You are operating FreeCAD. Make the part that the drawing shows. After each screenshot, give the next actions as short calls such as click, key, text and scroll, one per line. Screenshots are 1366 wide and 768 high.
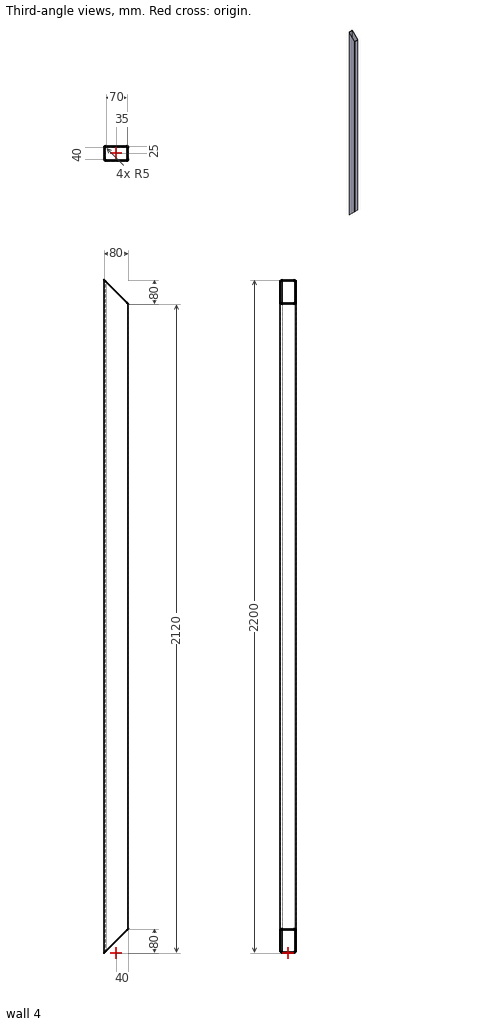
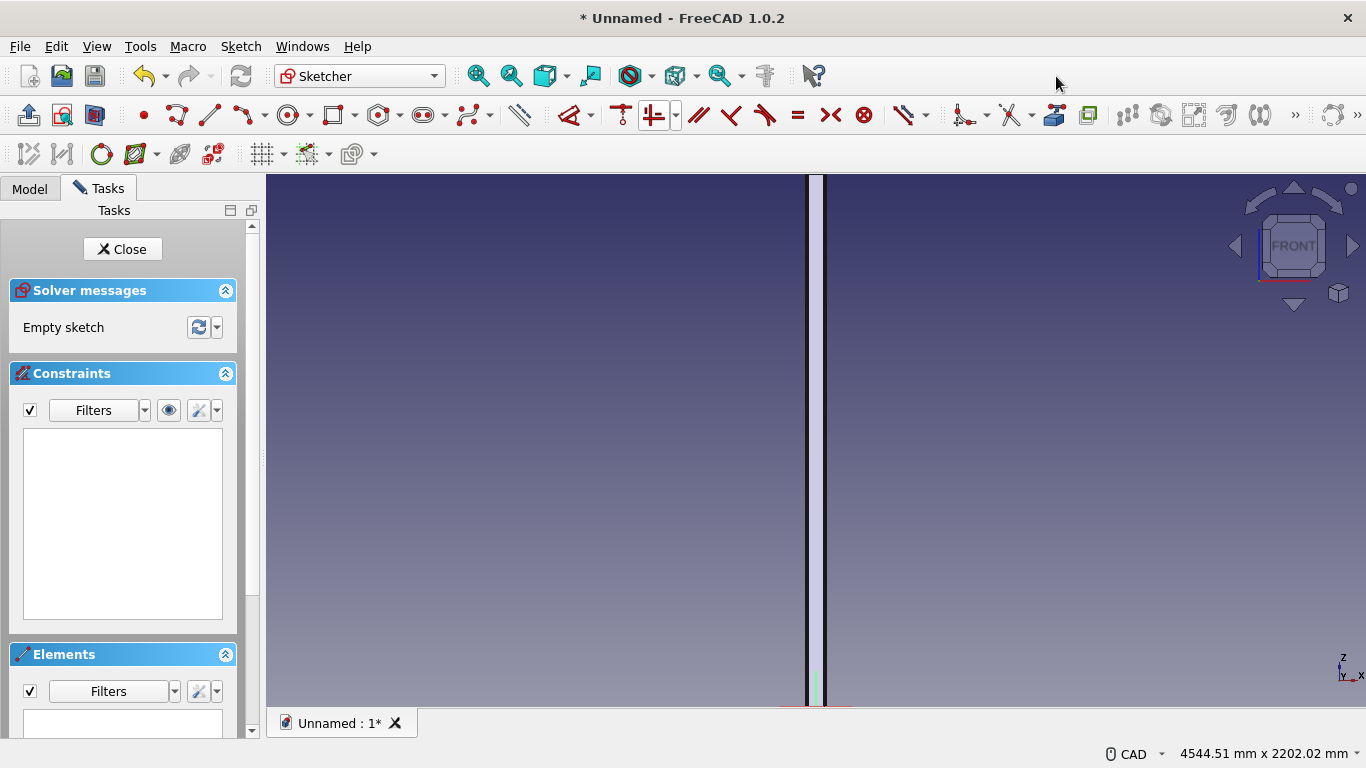
scroll(608, 441, down, 2)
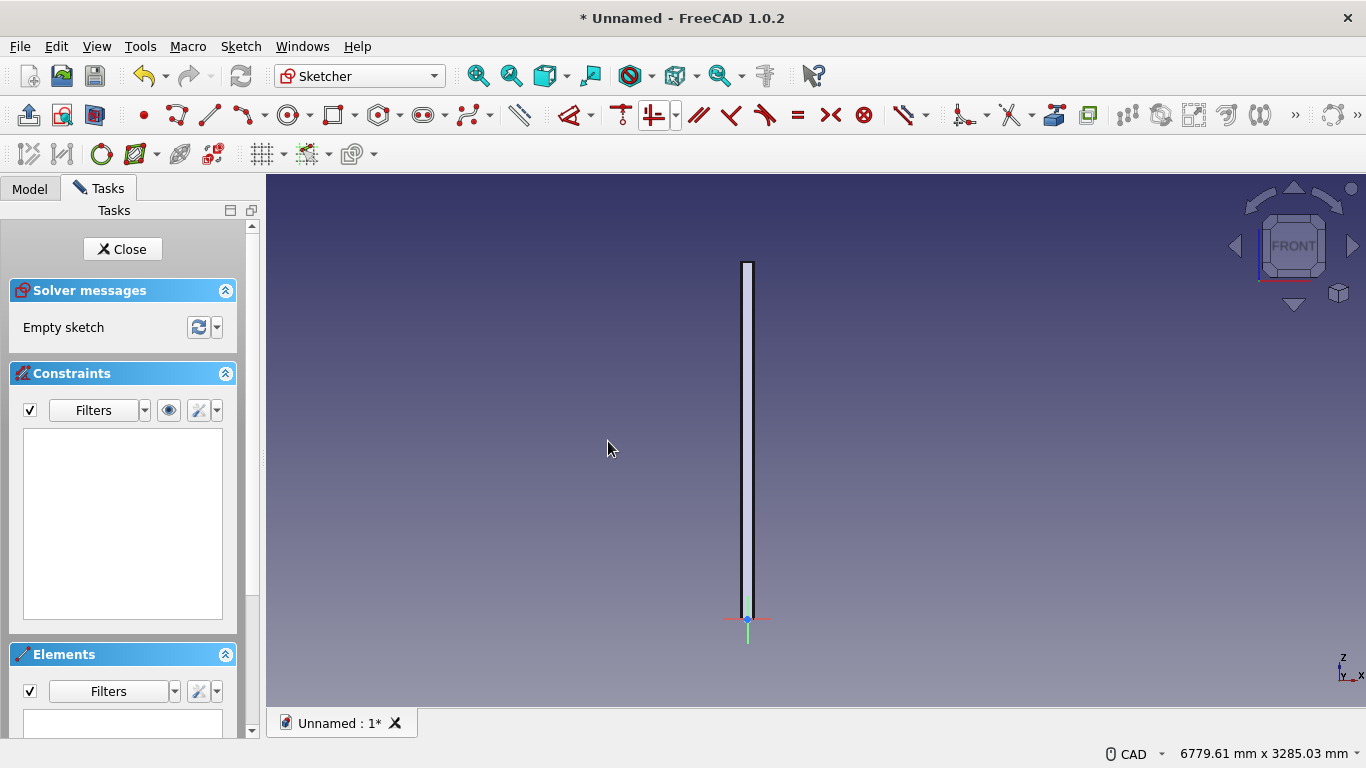
click(177, 116)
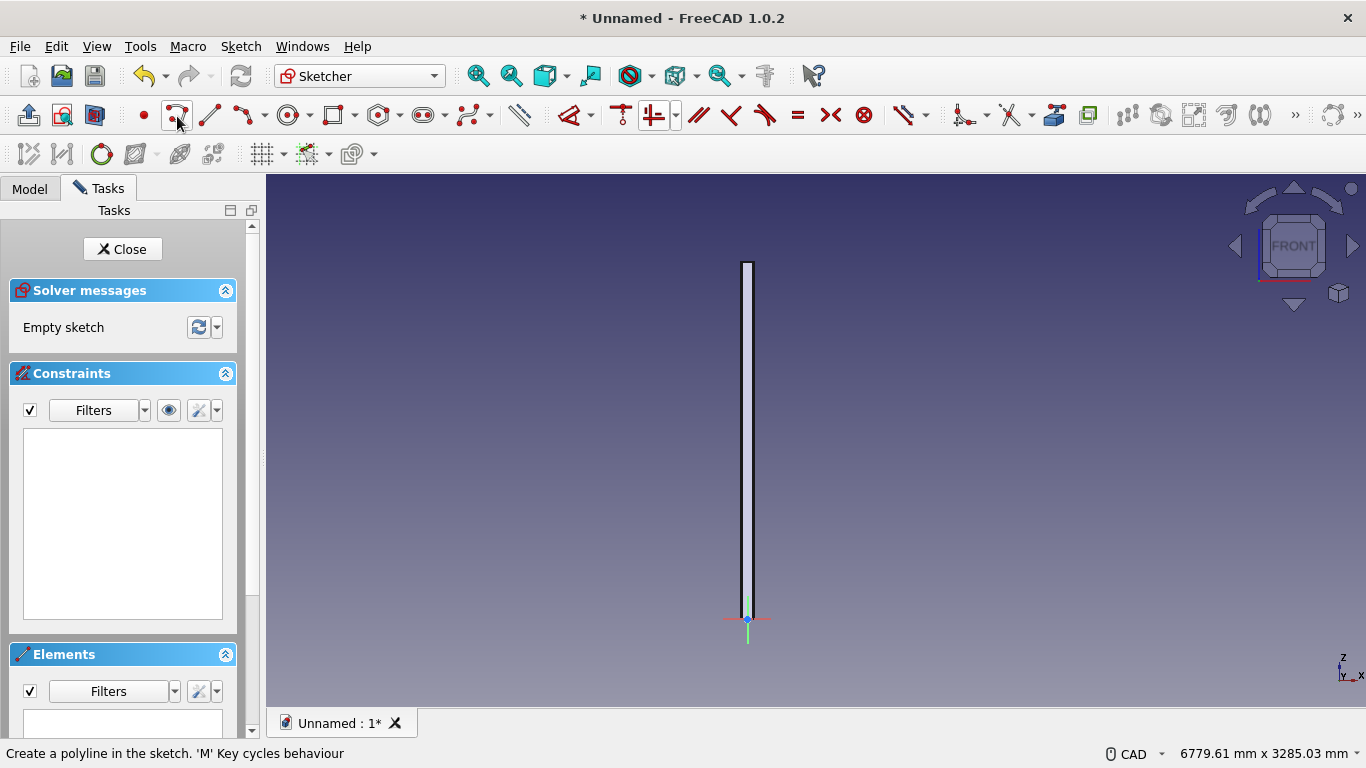
scroll(754, 275, up, 5)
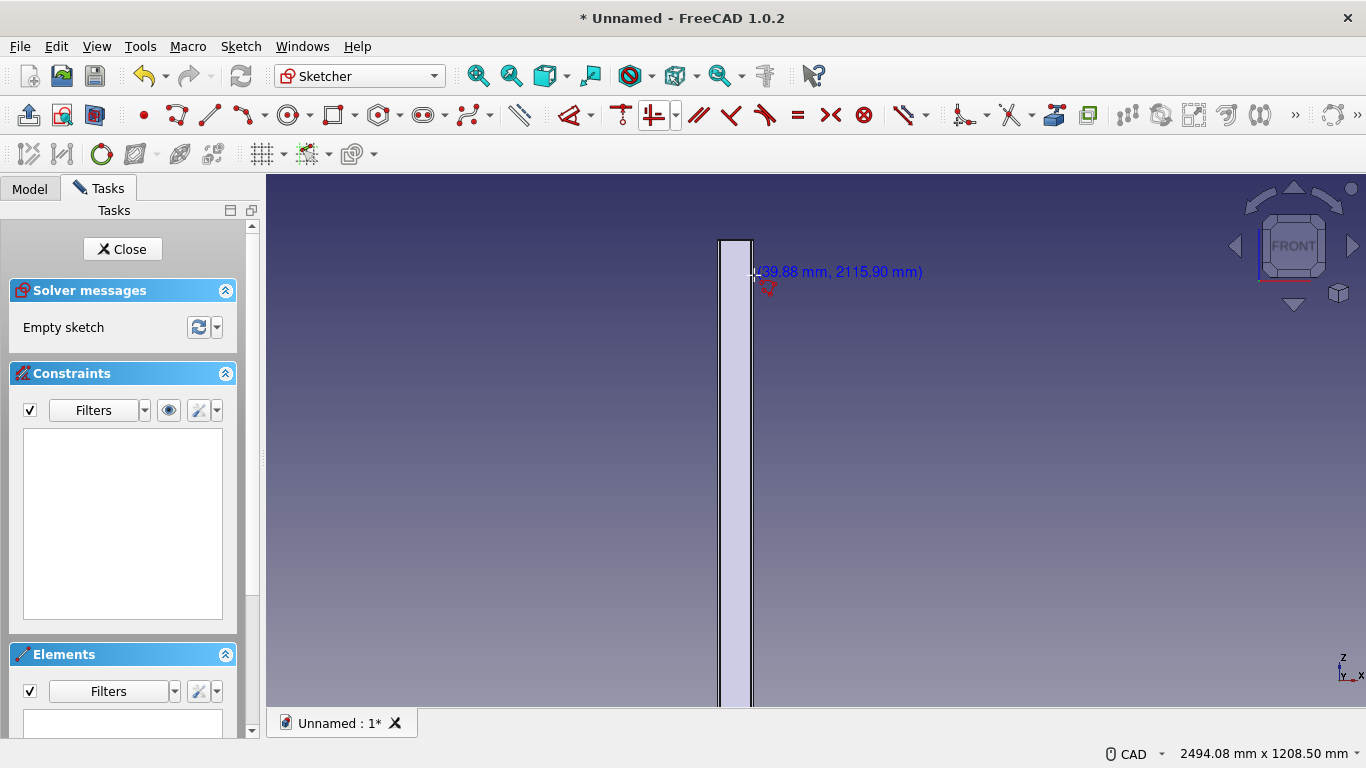
click(753, 276)
click(753, 240)
click(718, 240)
click(753, 277)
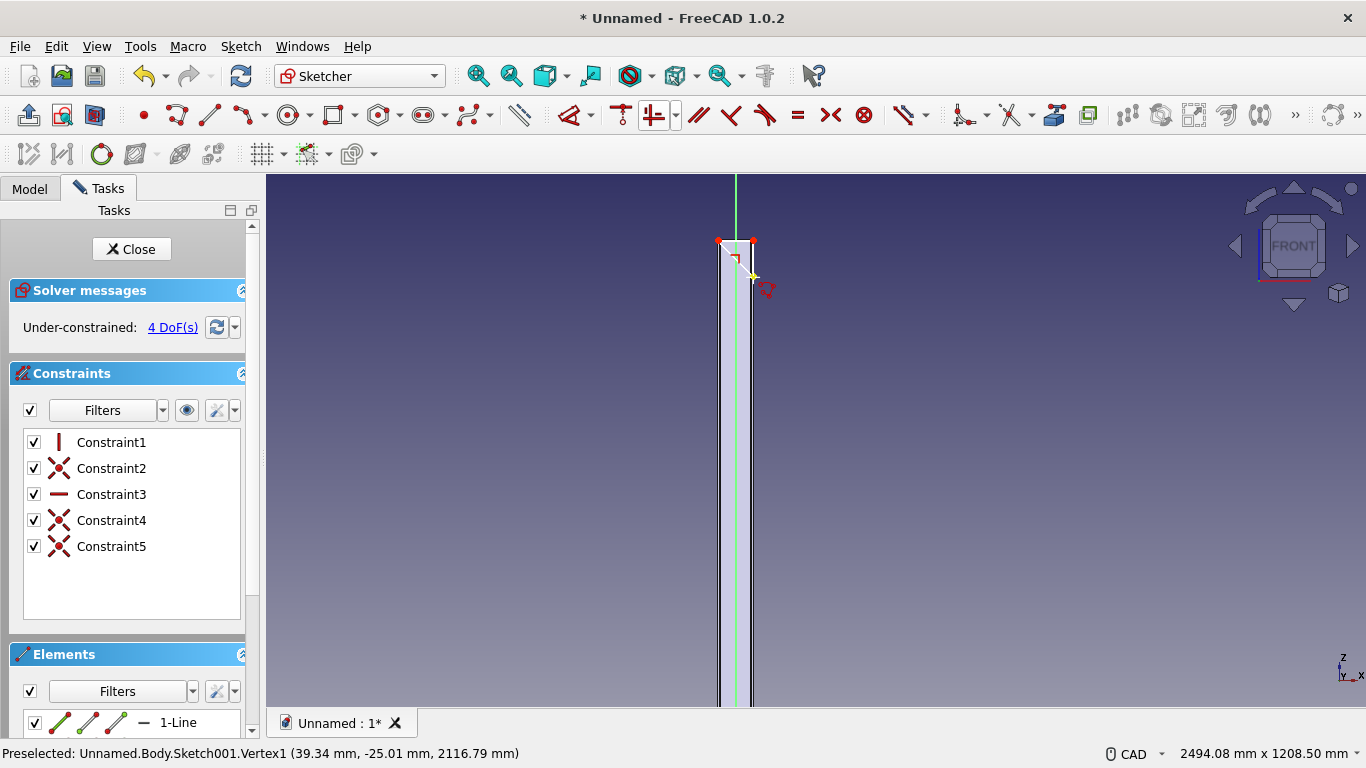
scroll(754, 275, down, 5)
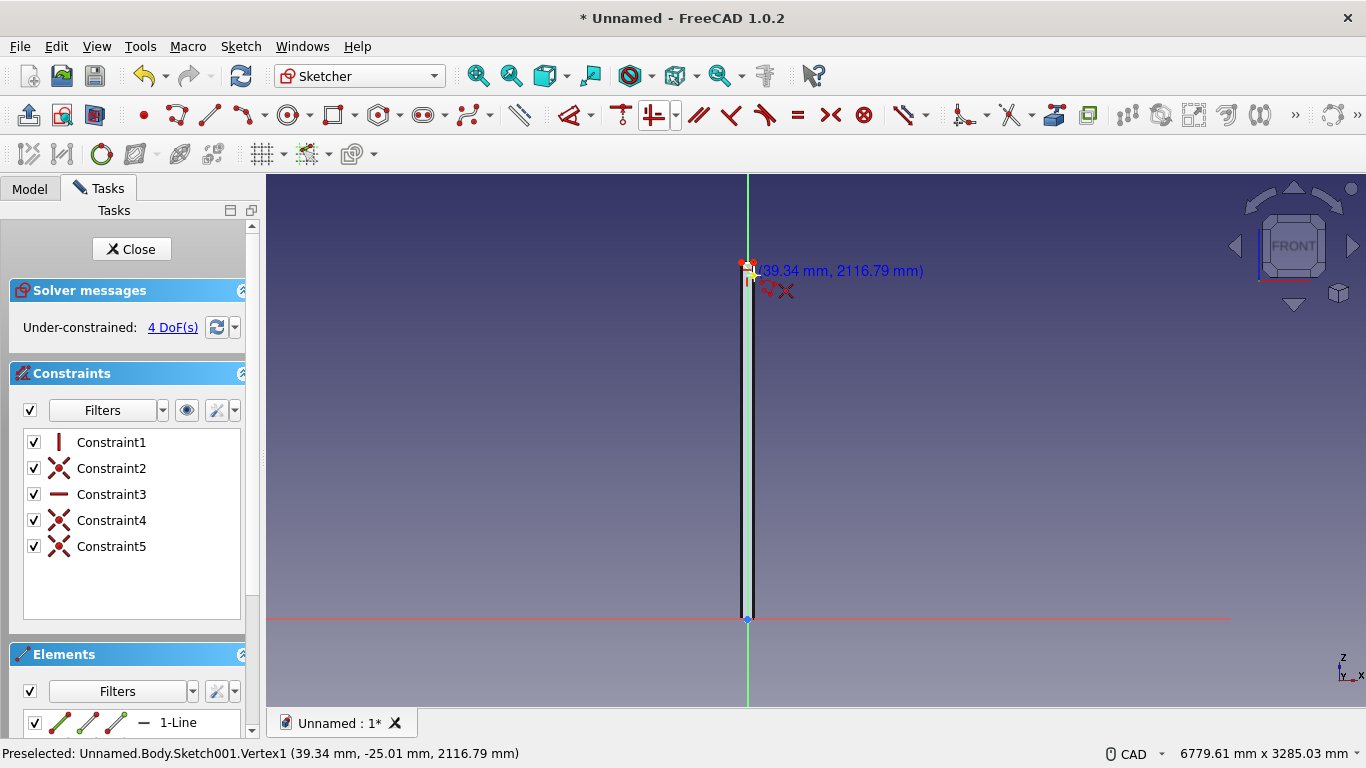
scroll(754, 619, up, 5)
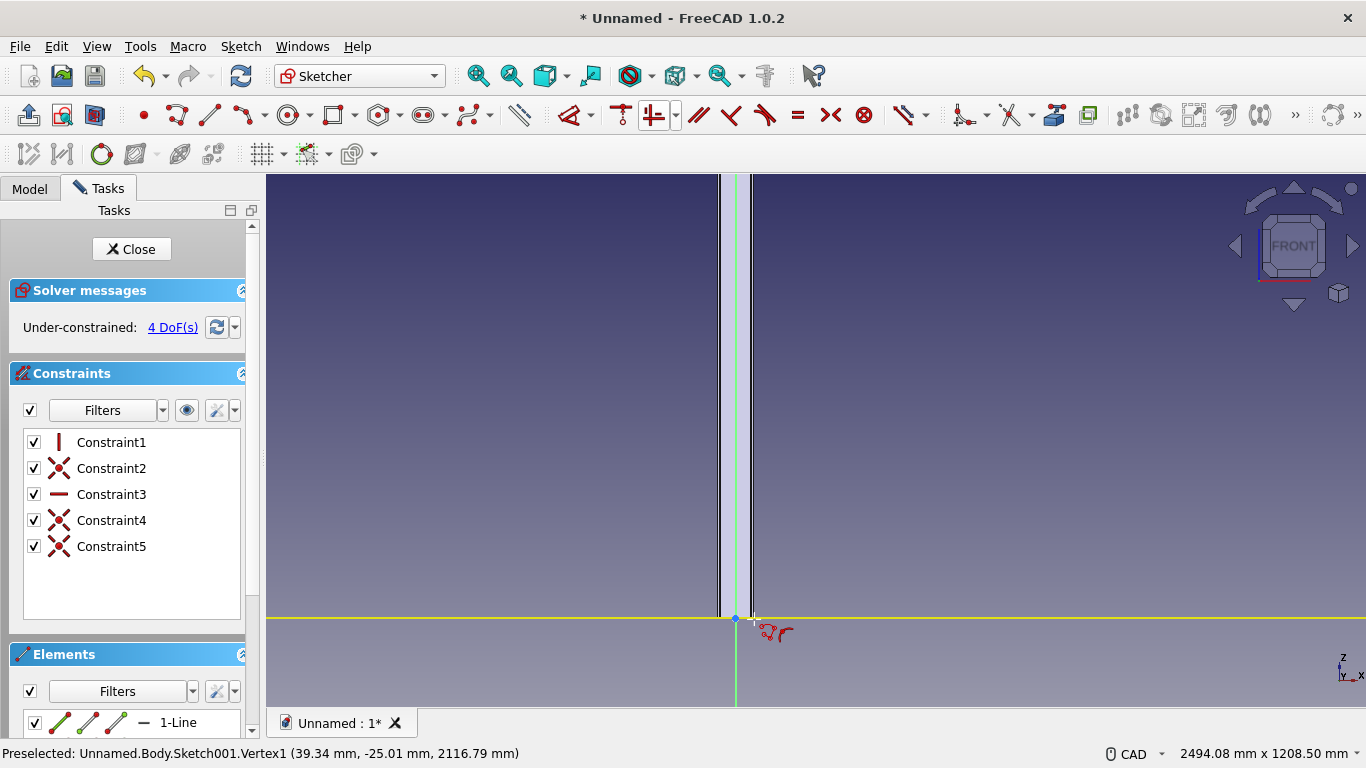
click(753, 618)
click(753, 583)
click(718, 609)
click(753, 618)
key(Escape)
key(Escape)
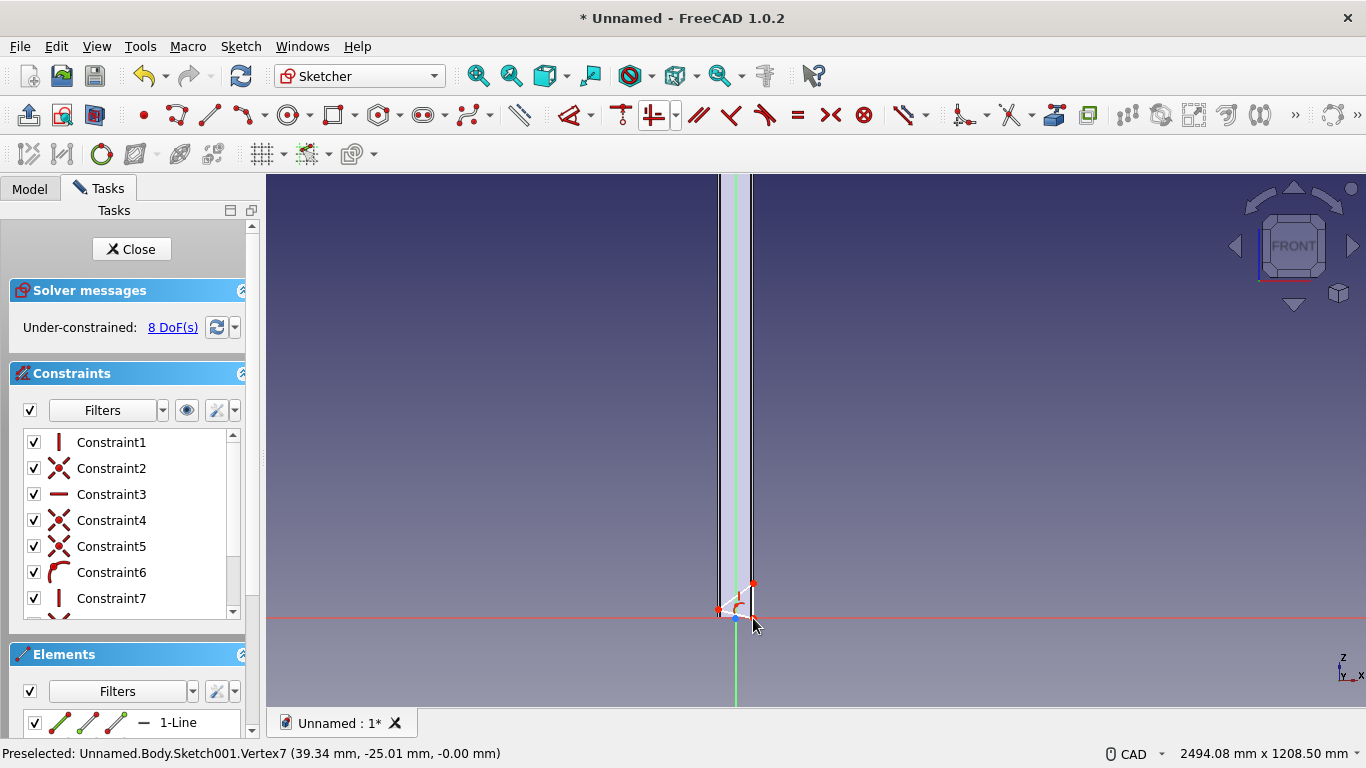
click(746, 617)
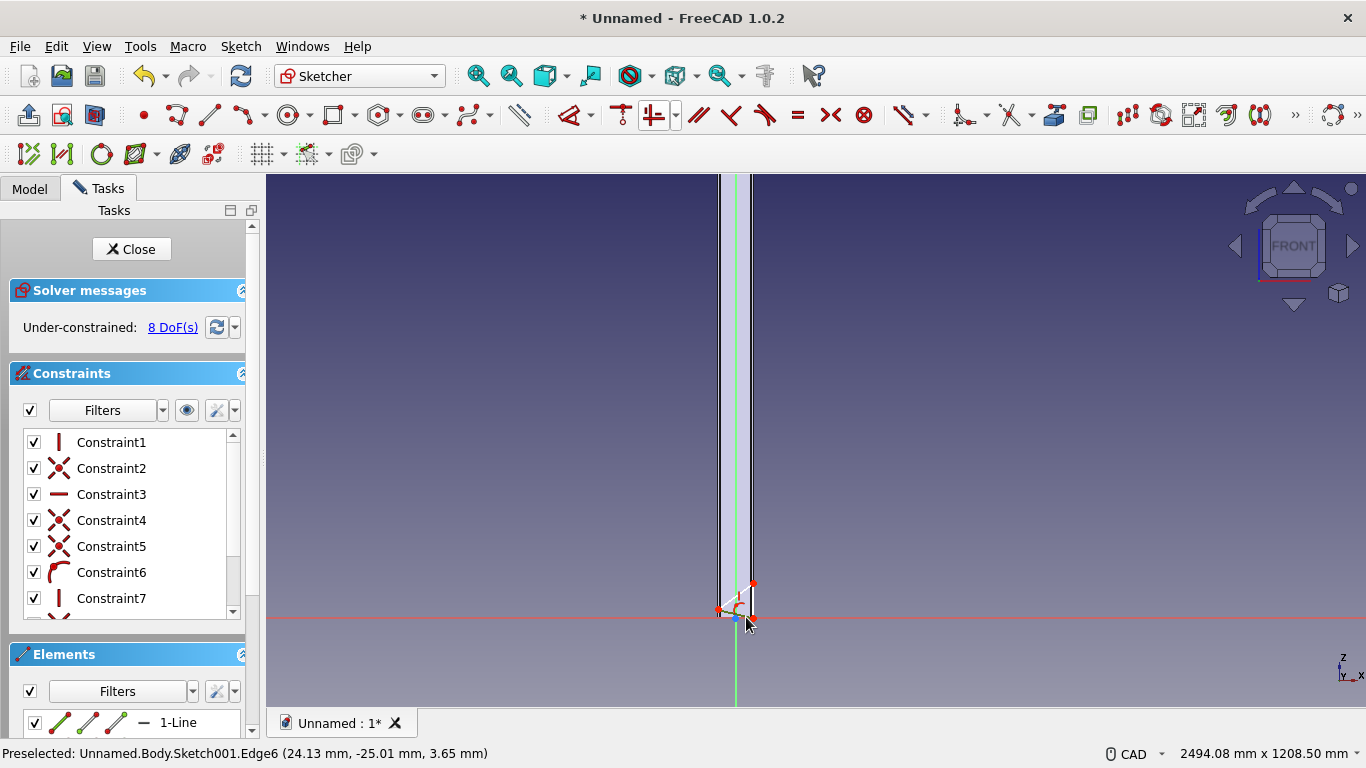
click(676, 116)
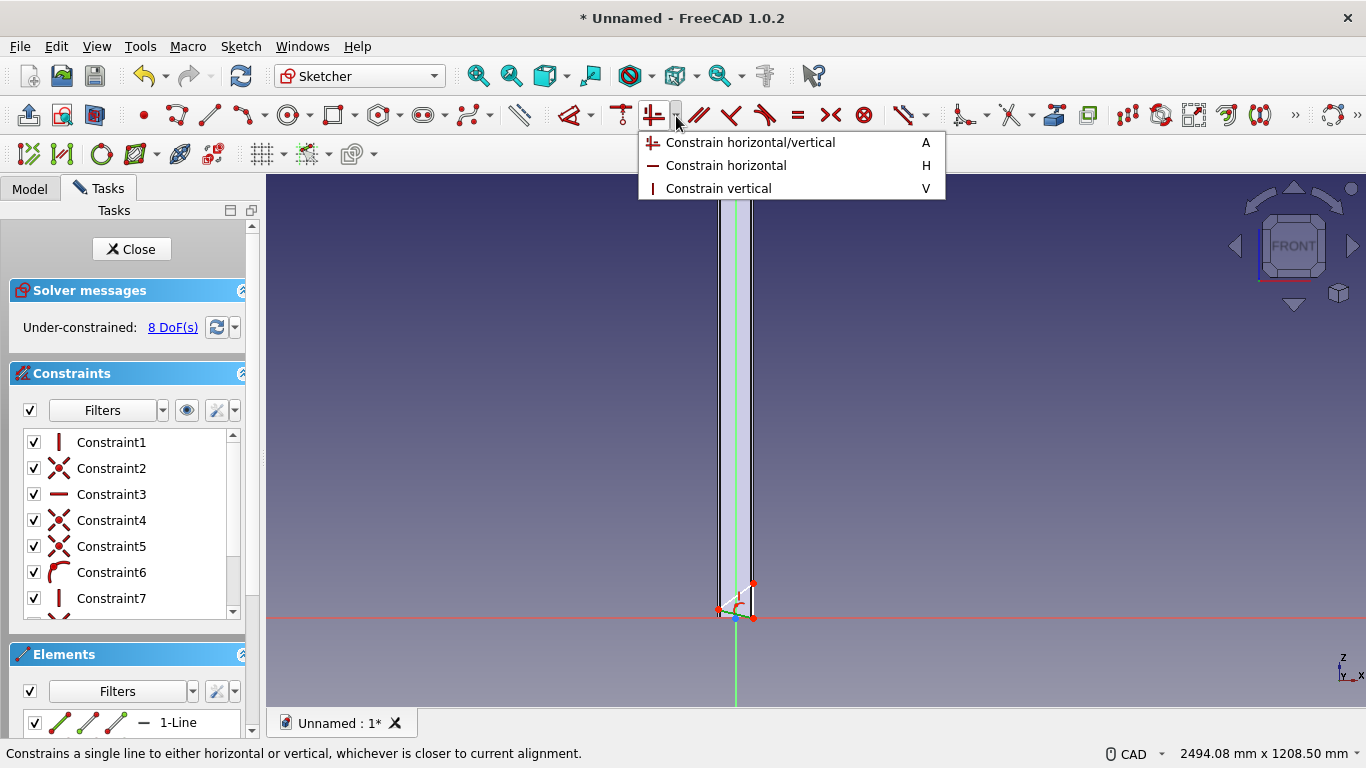
click(792, 166)